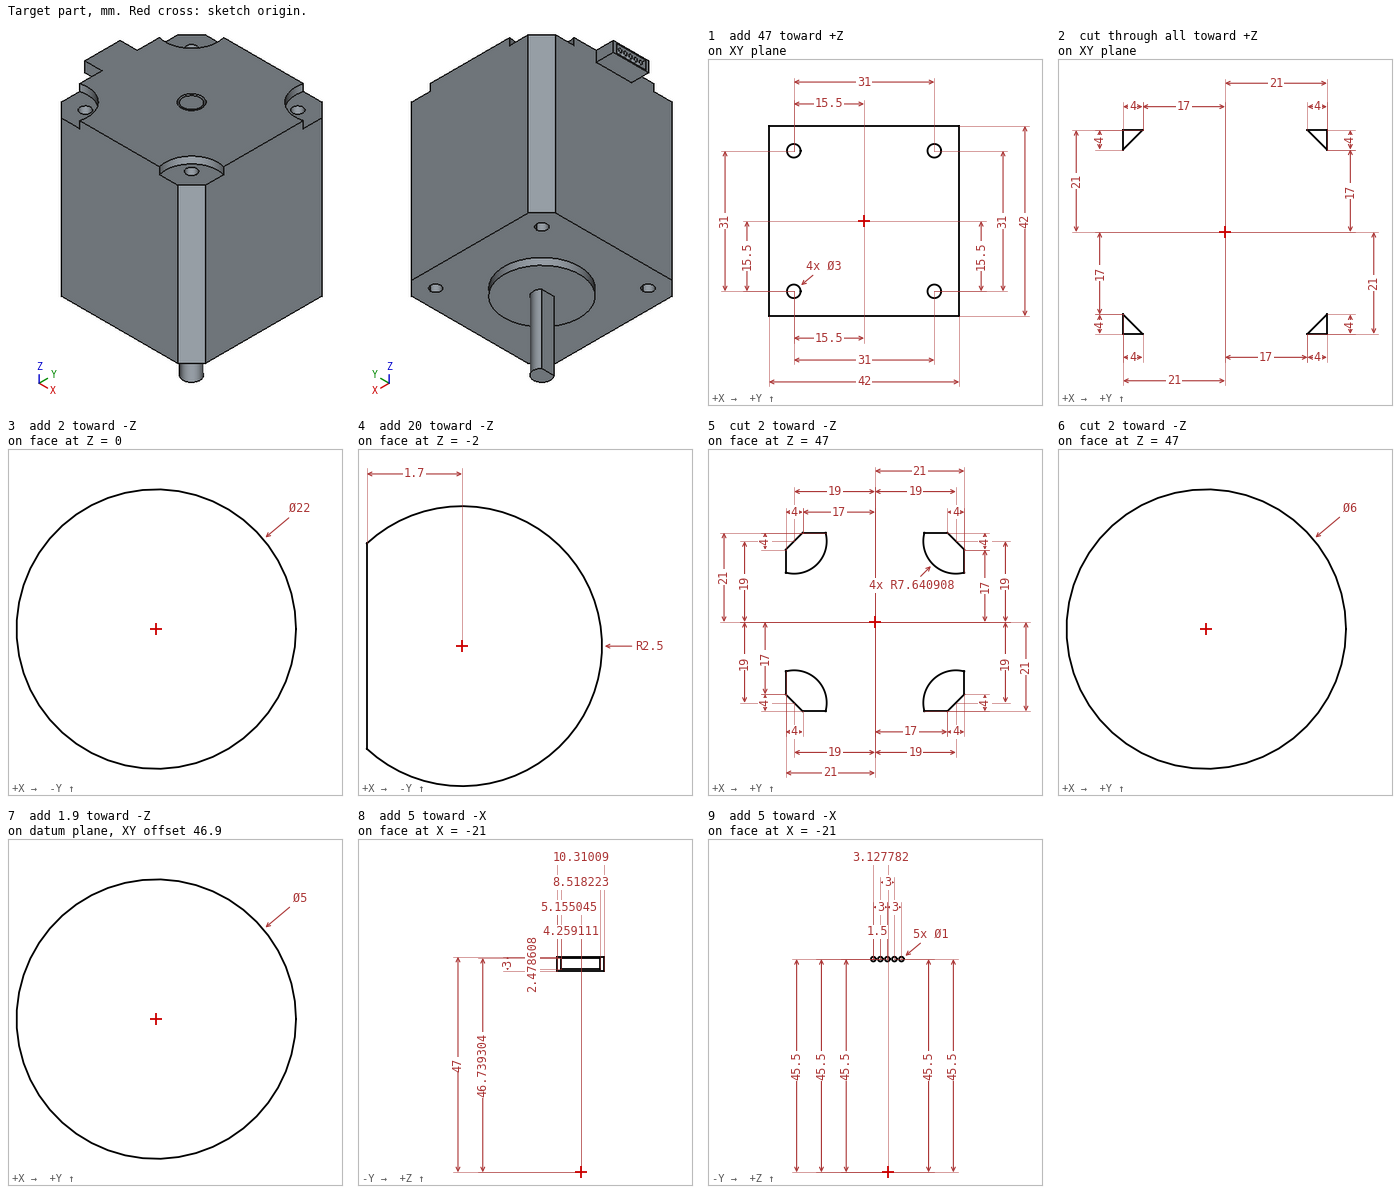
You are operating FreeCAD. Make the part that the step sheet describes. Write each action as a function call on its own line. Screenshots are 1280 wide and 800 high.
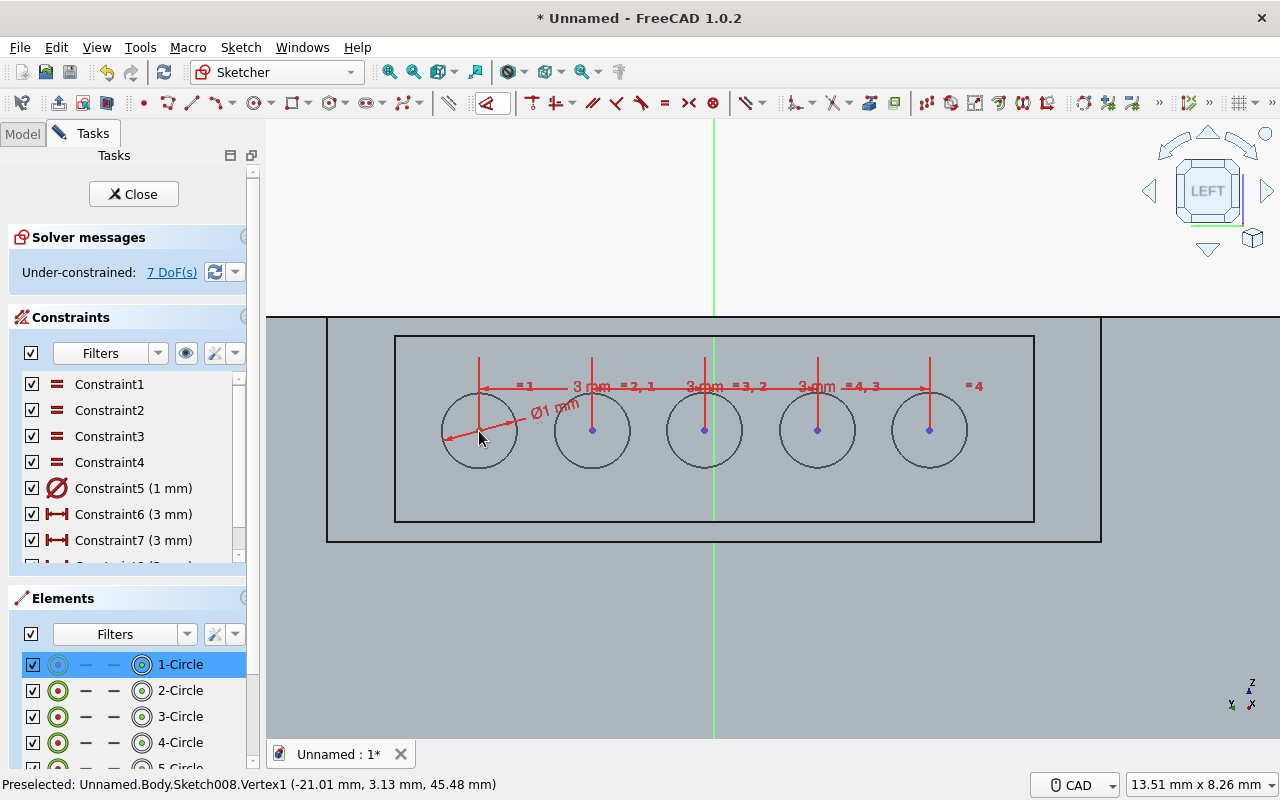
click(504, 104)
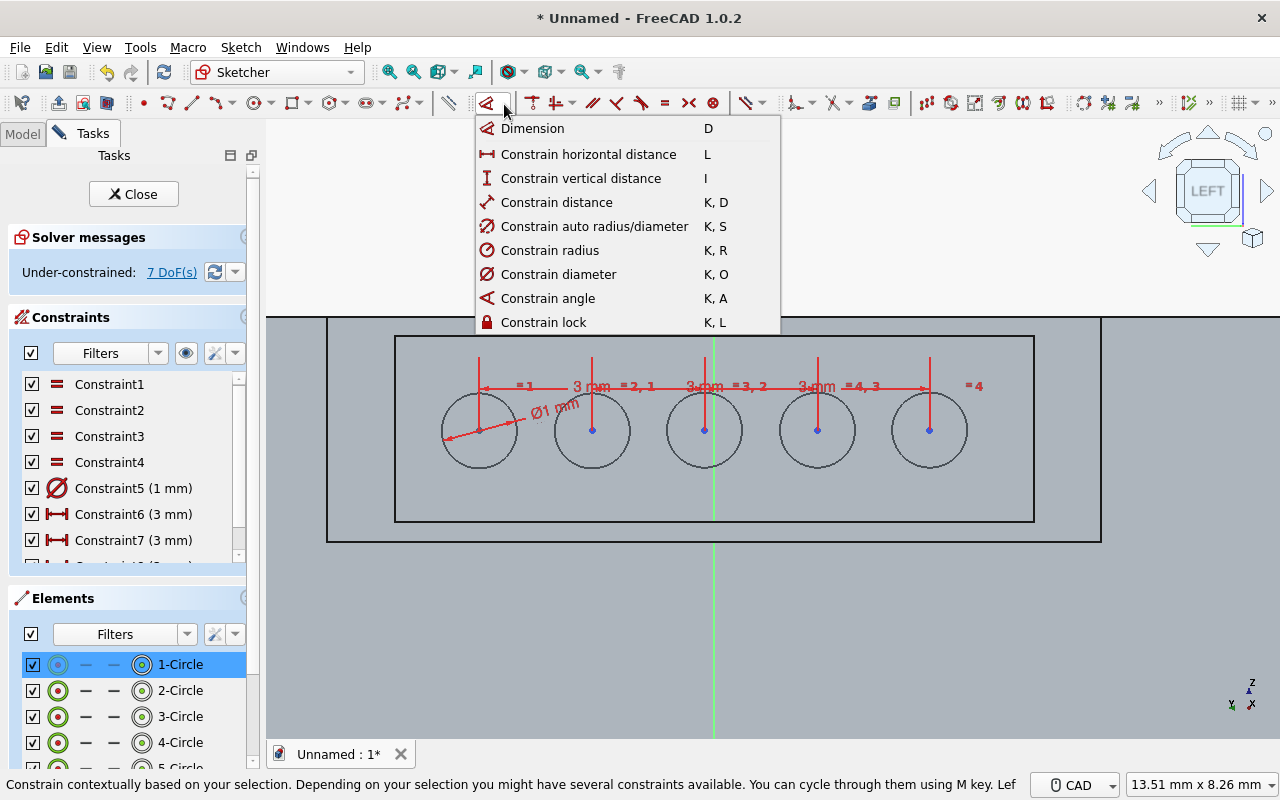
click(628, 178)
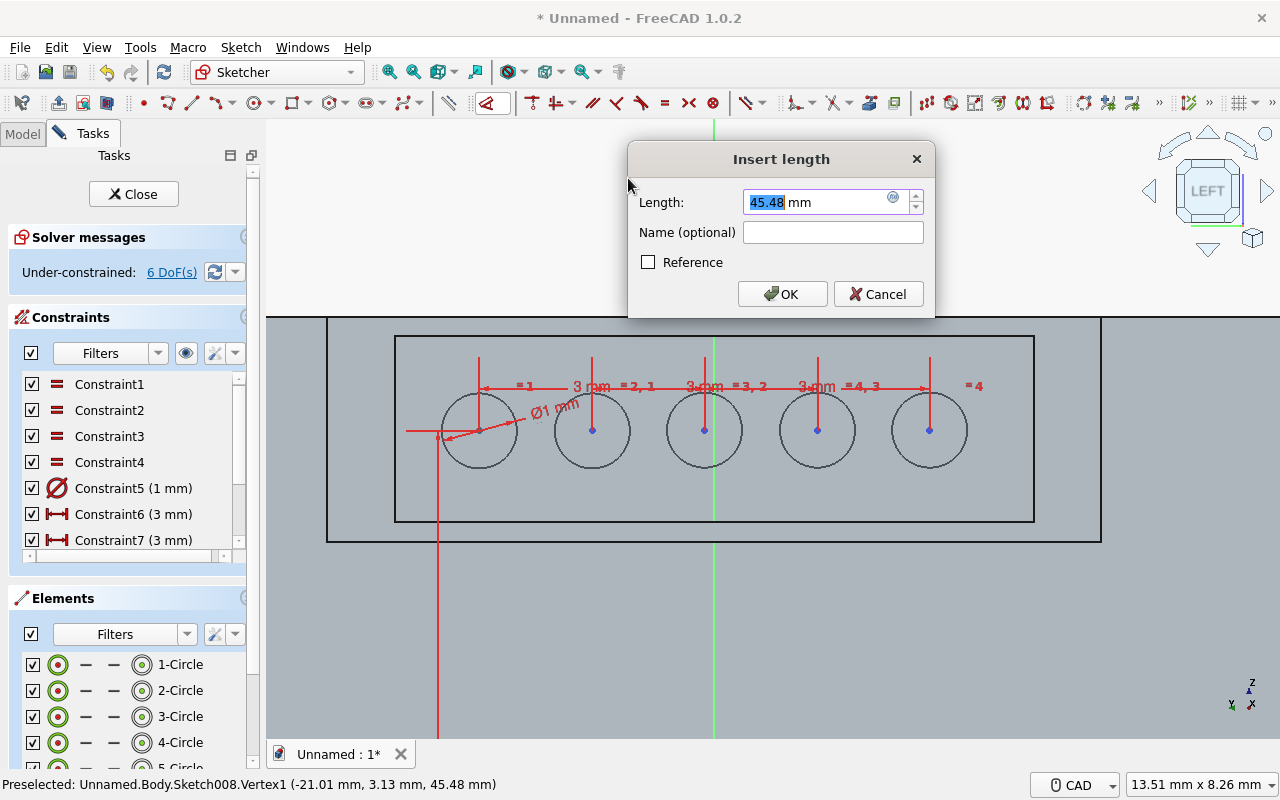
text(45.5)
key(Return)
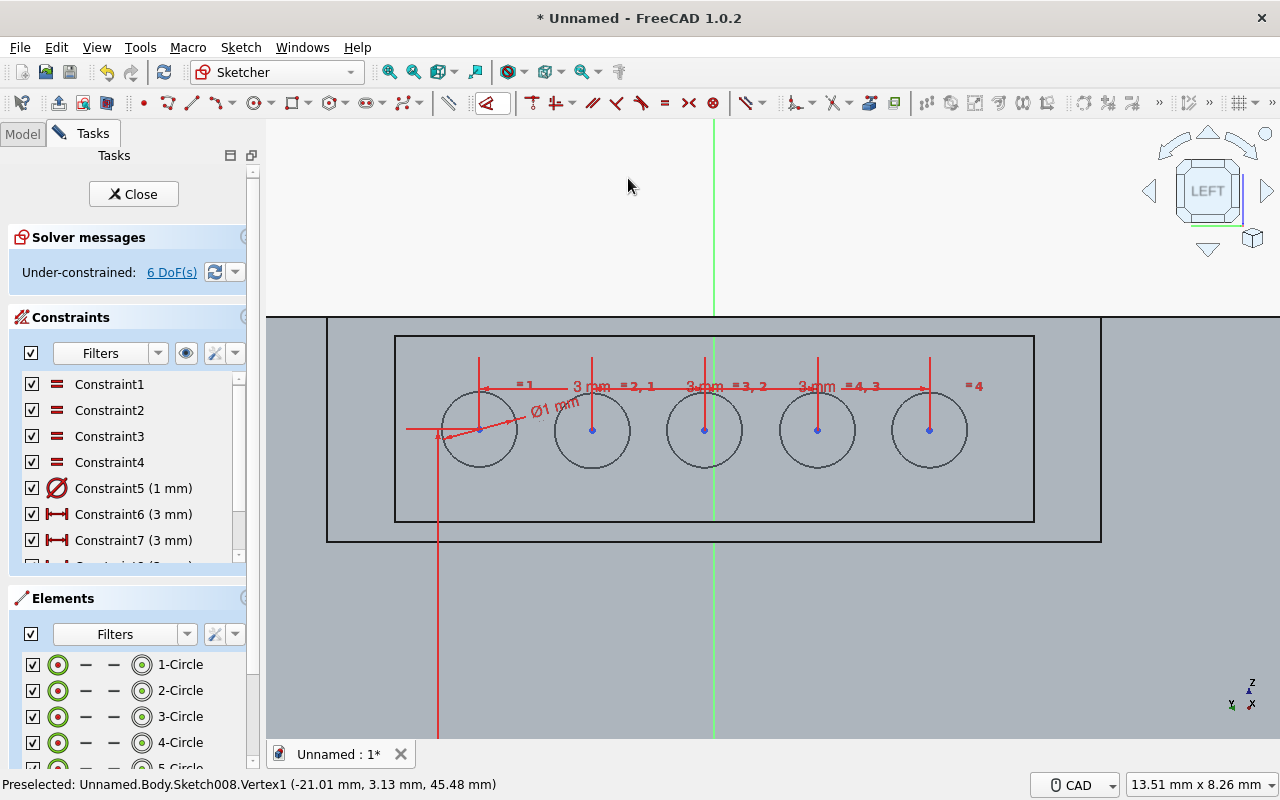
click(592, 431)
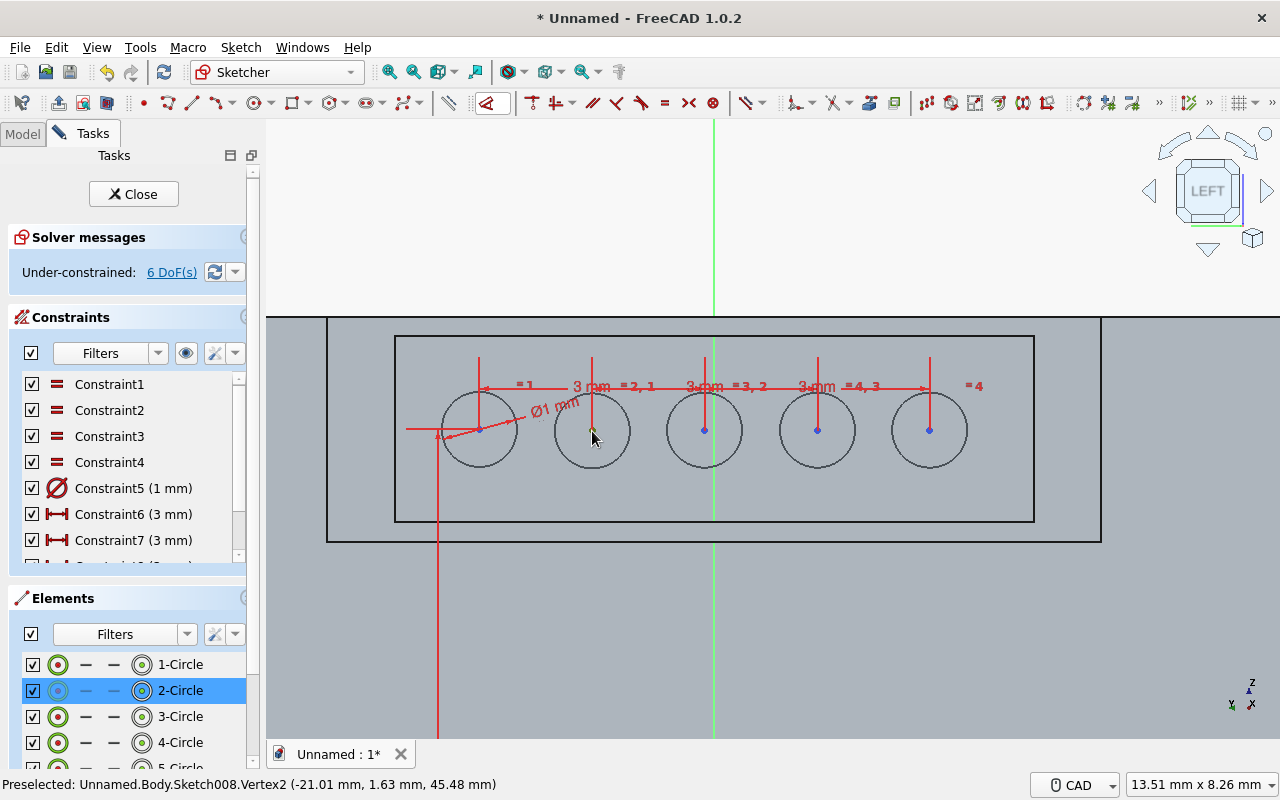
click(504, 104)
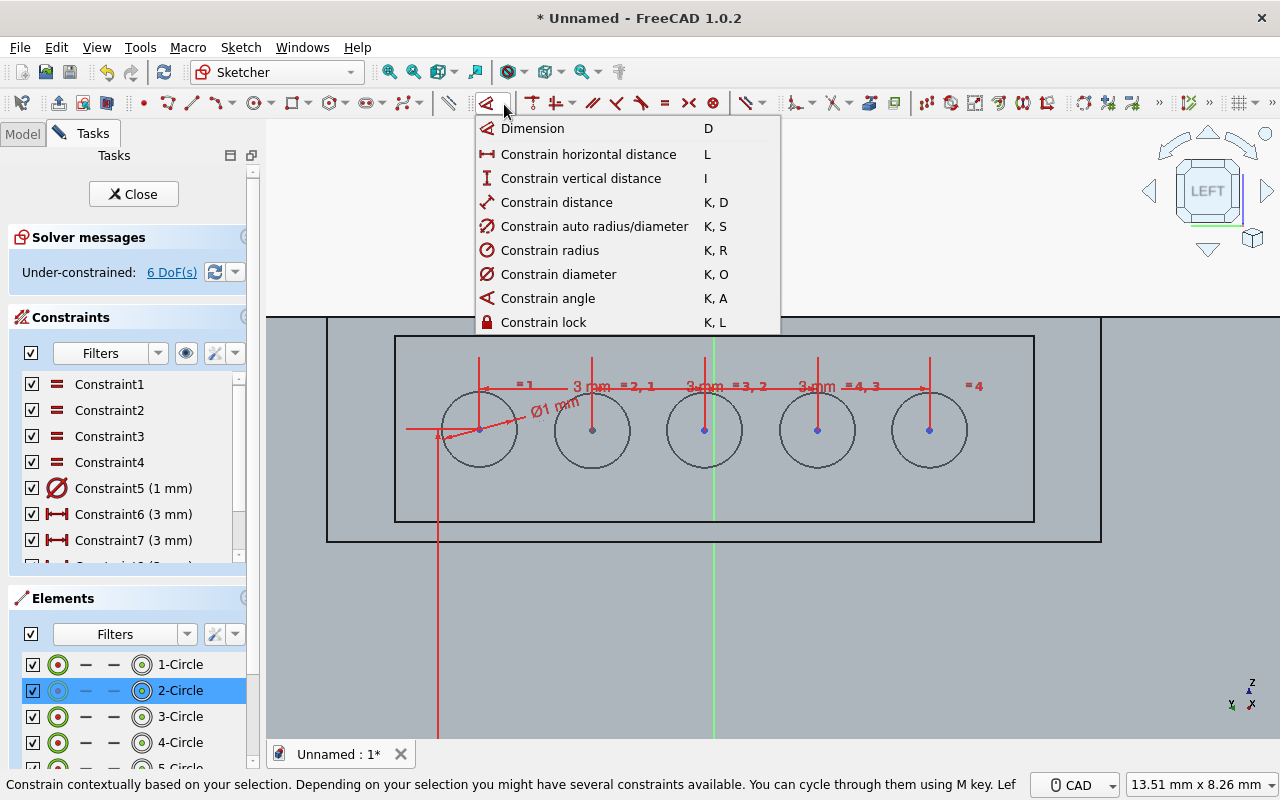
click(628, 178)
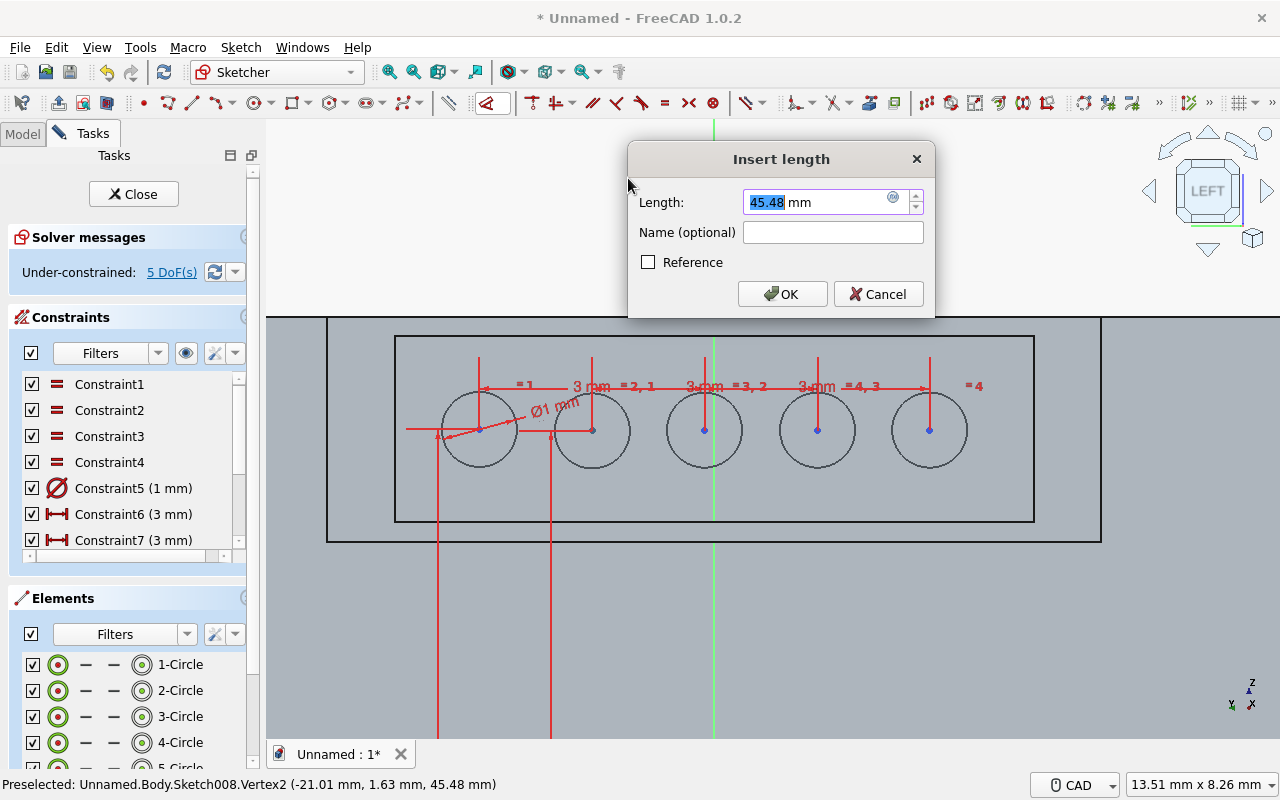
text(45.5)
key(Return)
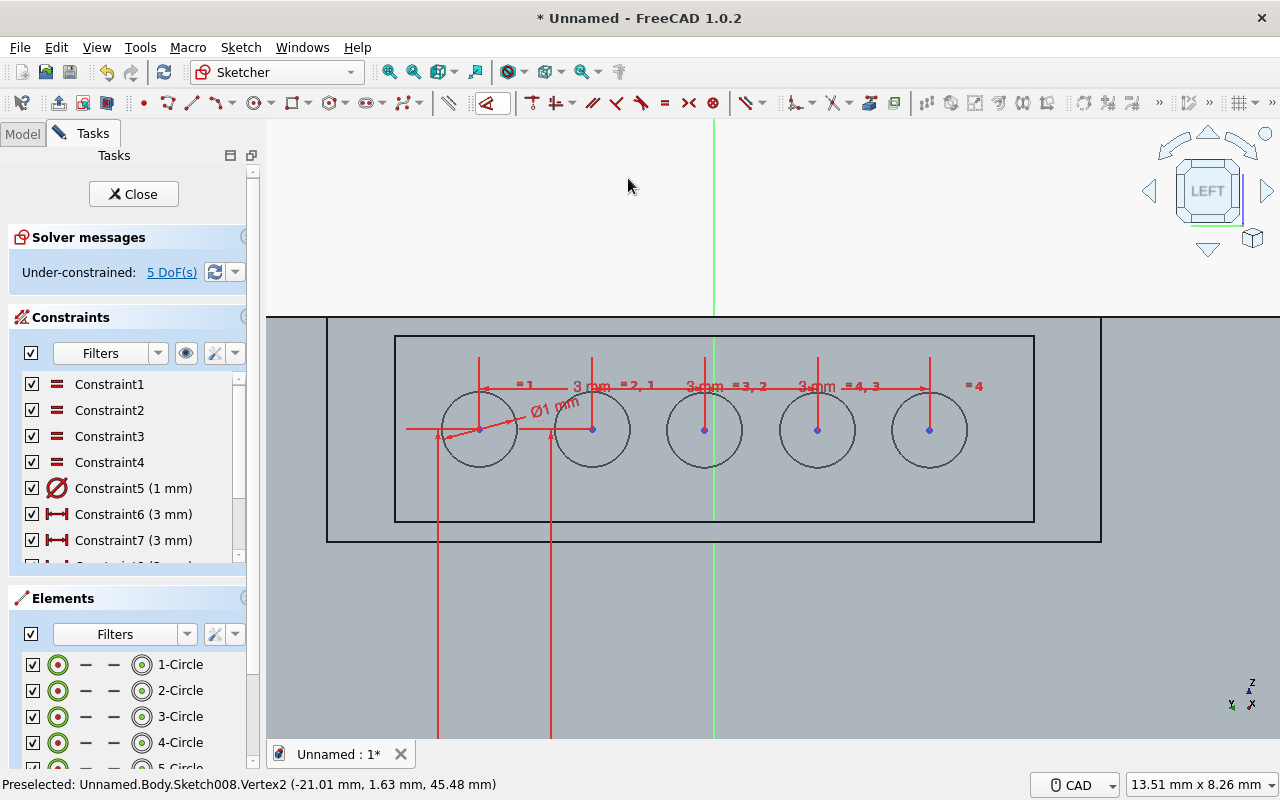
click(705, 430)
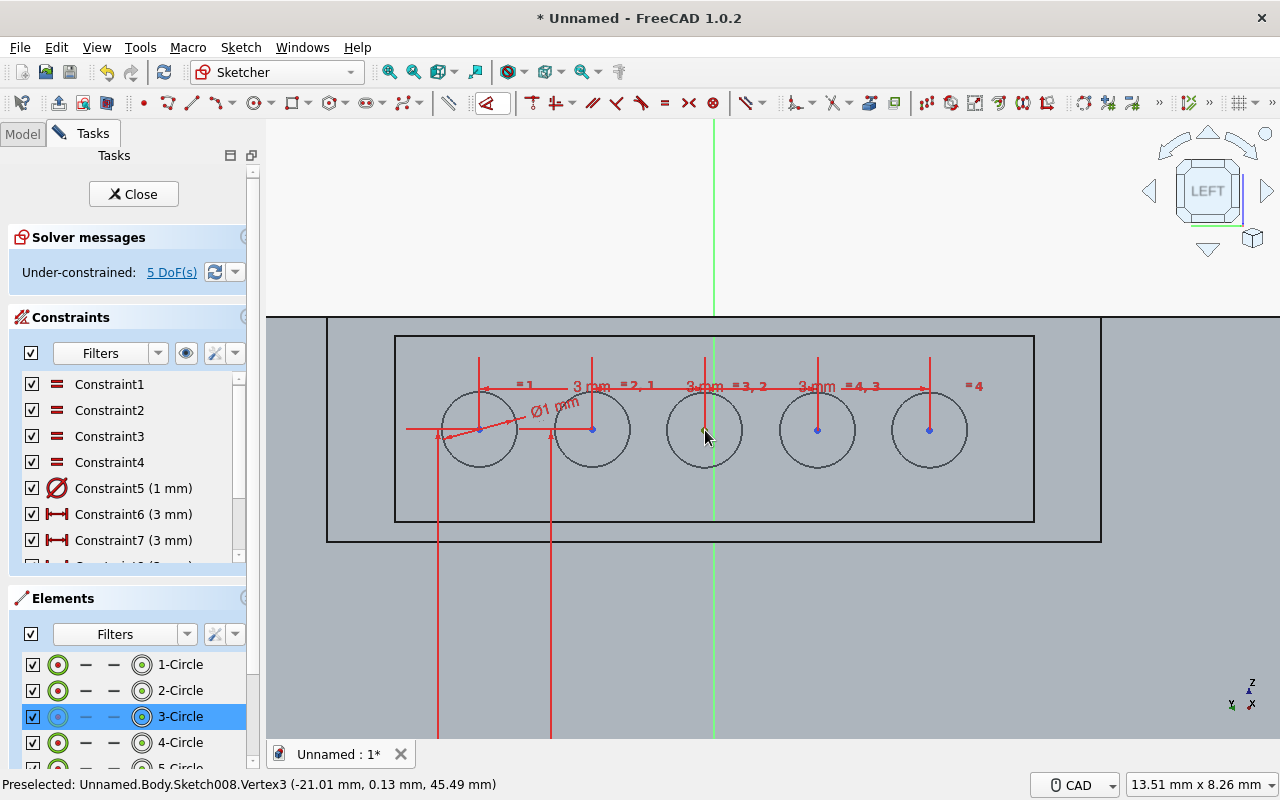
key(i)